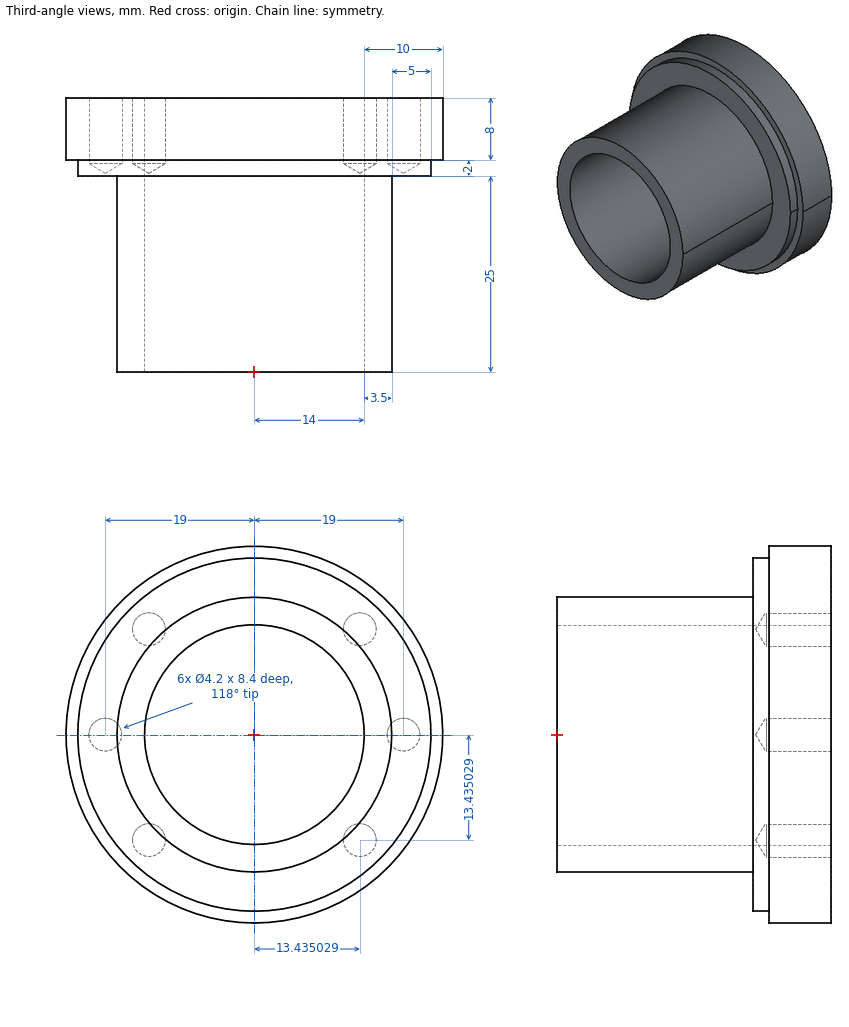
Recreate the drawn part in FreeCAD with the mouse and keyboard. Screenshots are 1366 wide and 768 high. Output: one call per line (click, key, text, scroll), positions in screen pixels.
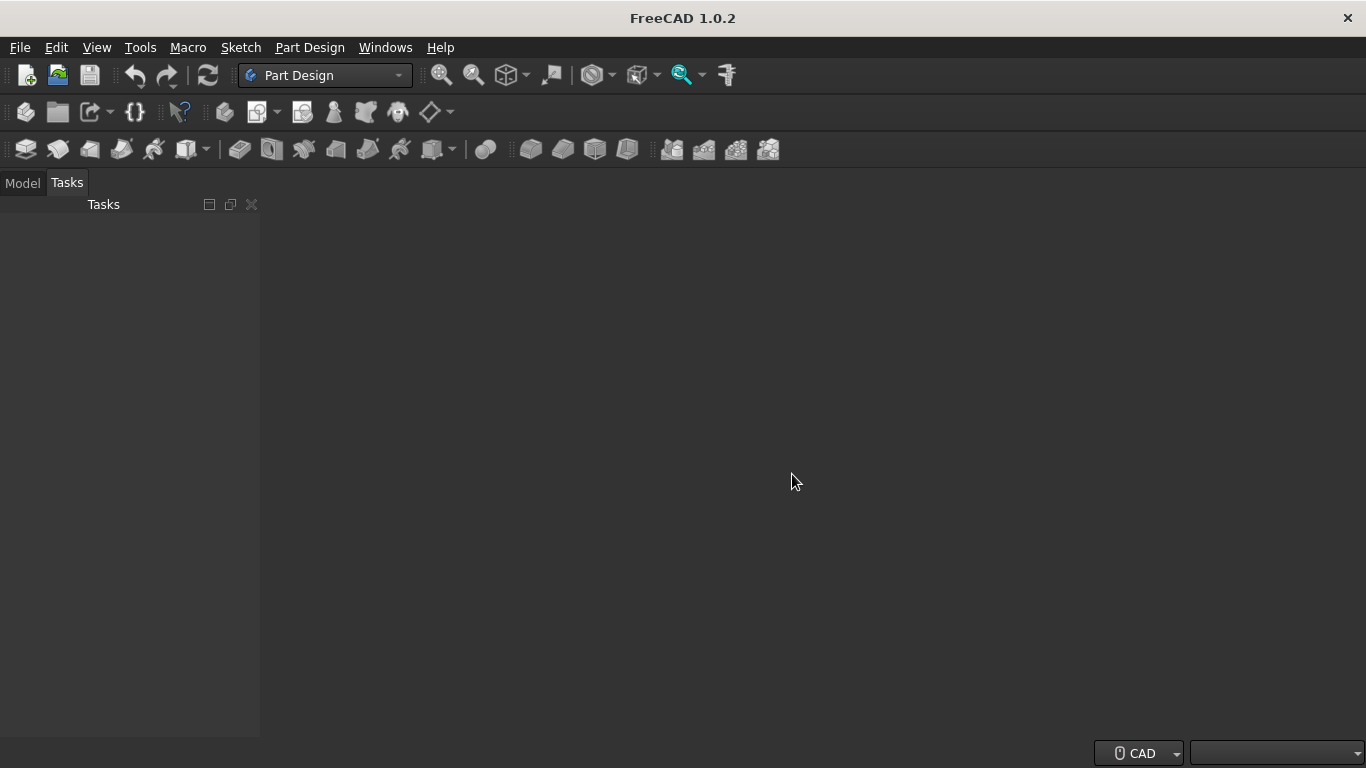
click(26, 76)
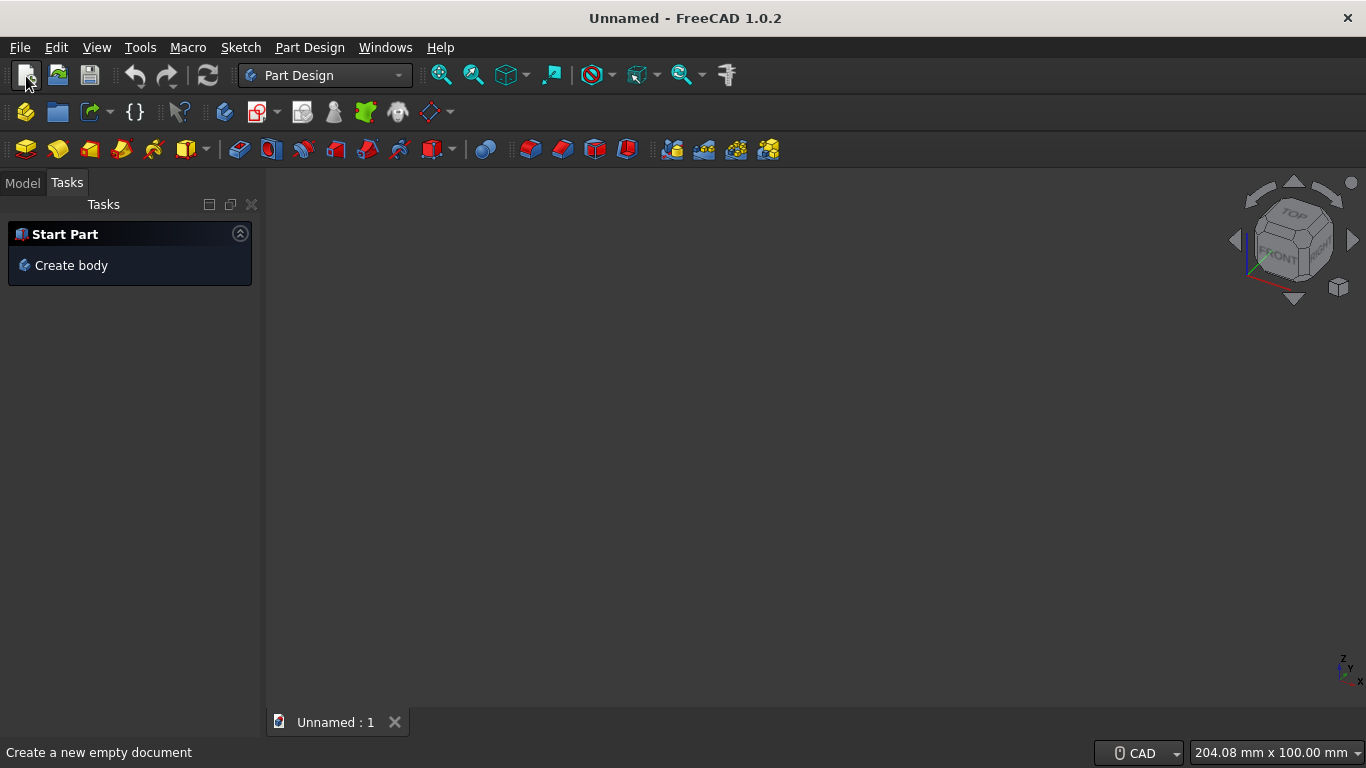
click(258, 112)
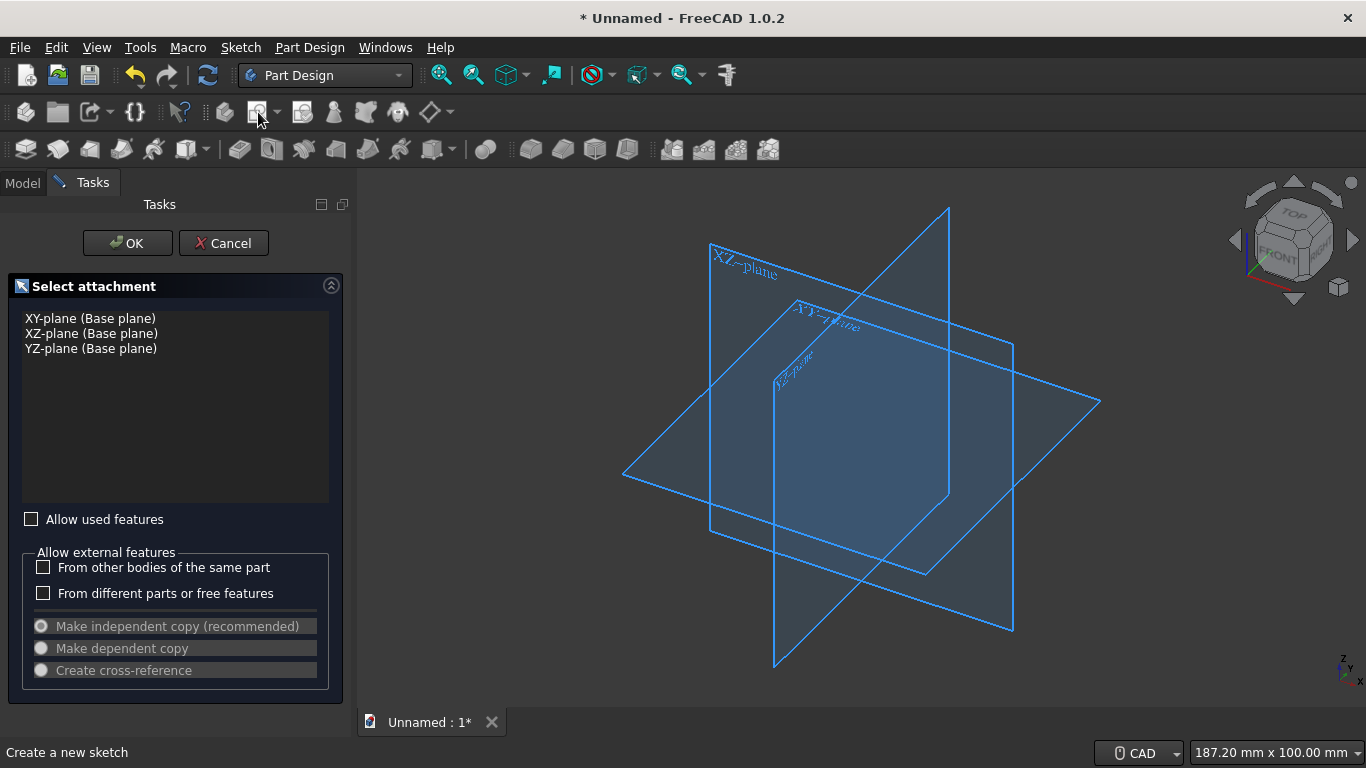
click(82, 318)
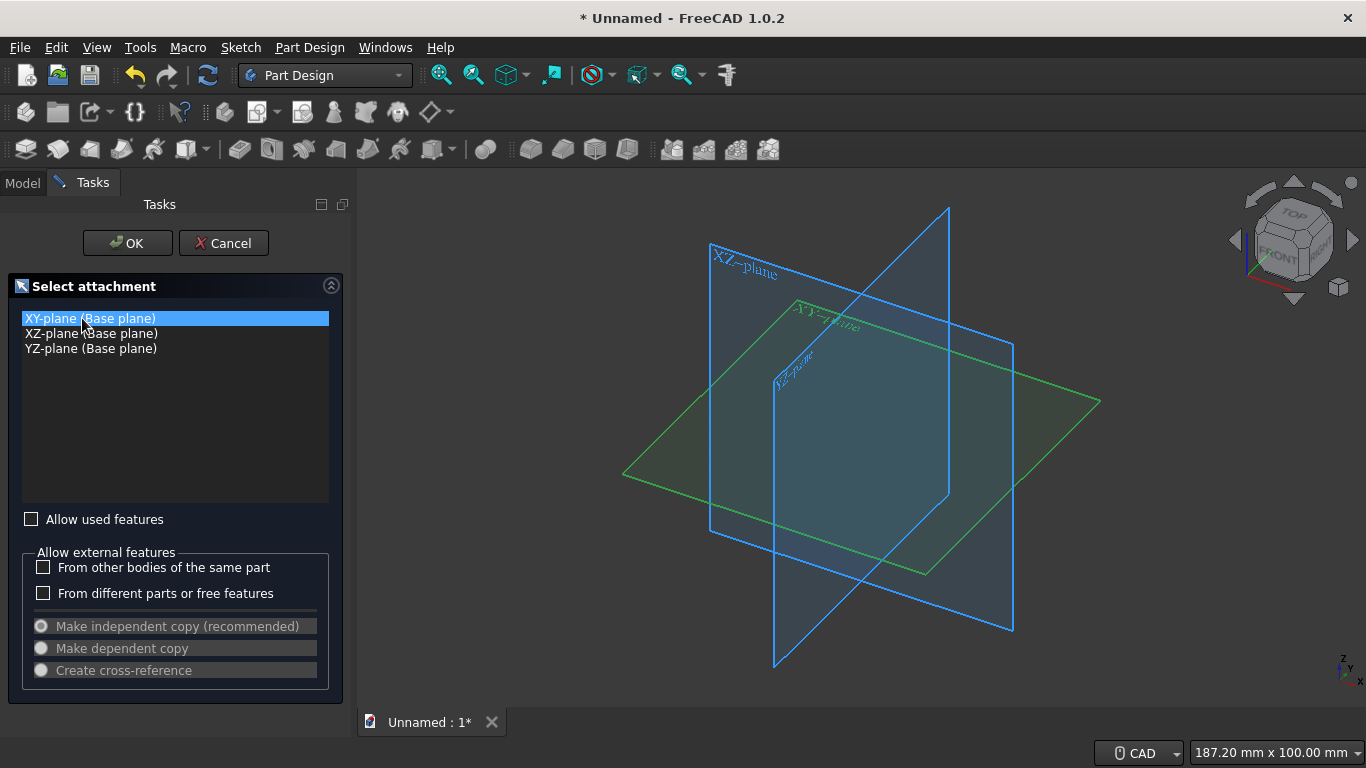
click(128, 243)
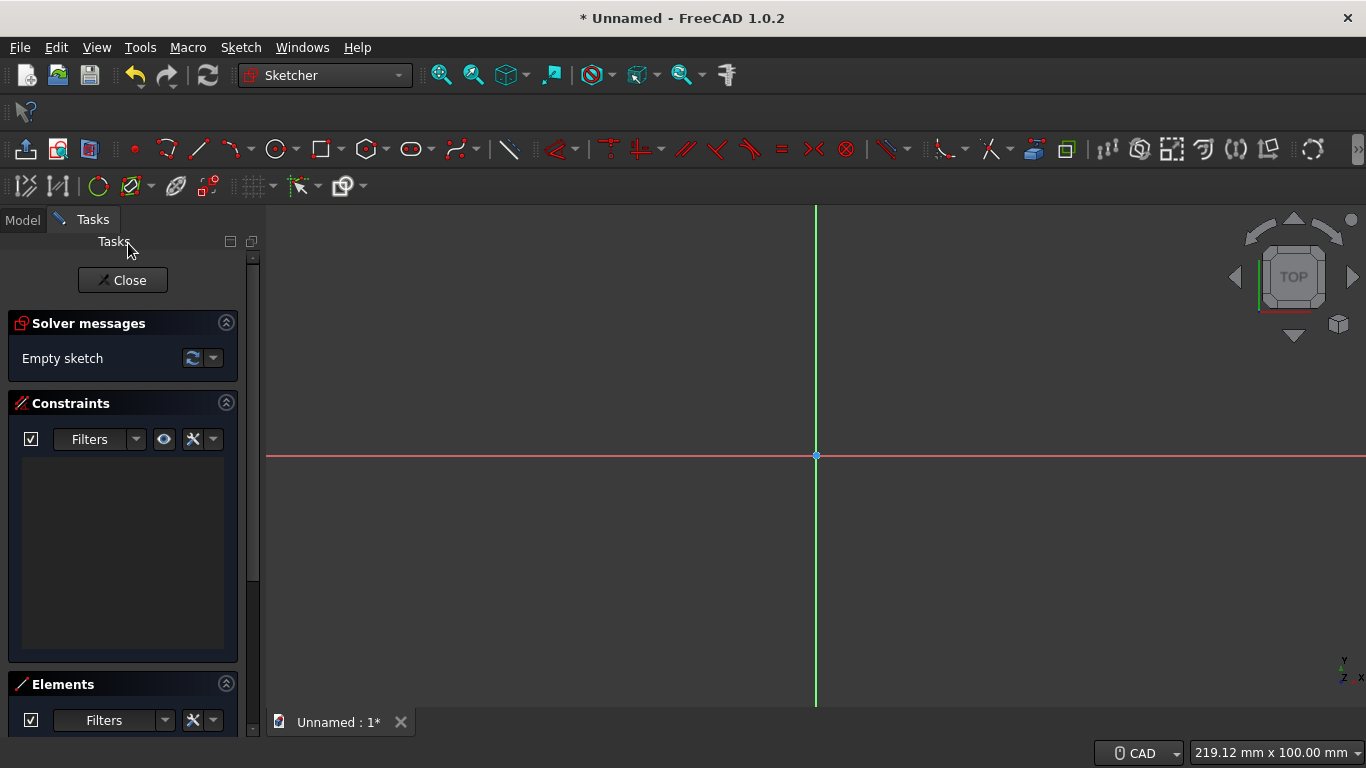
scroll(1033, 261, up, 3)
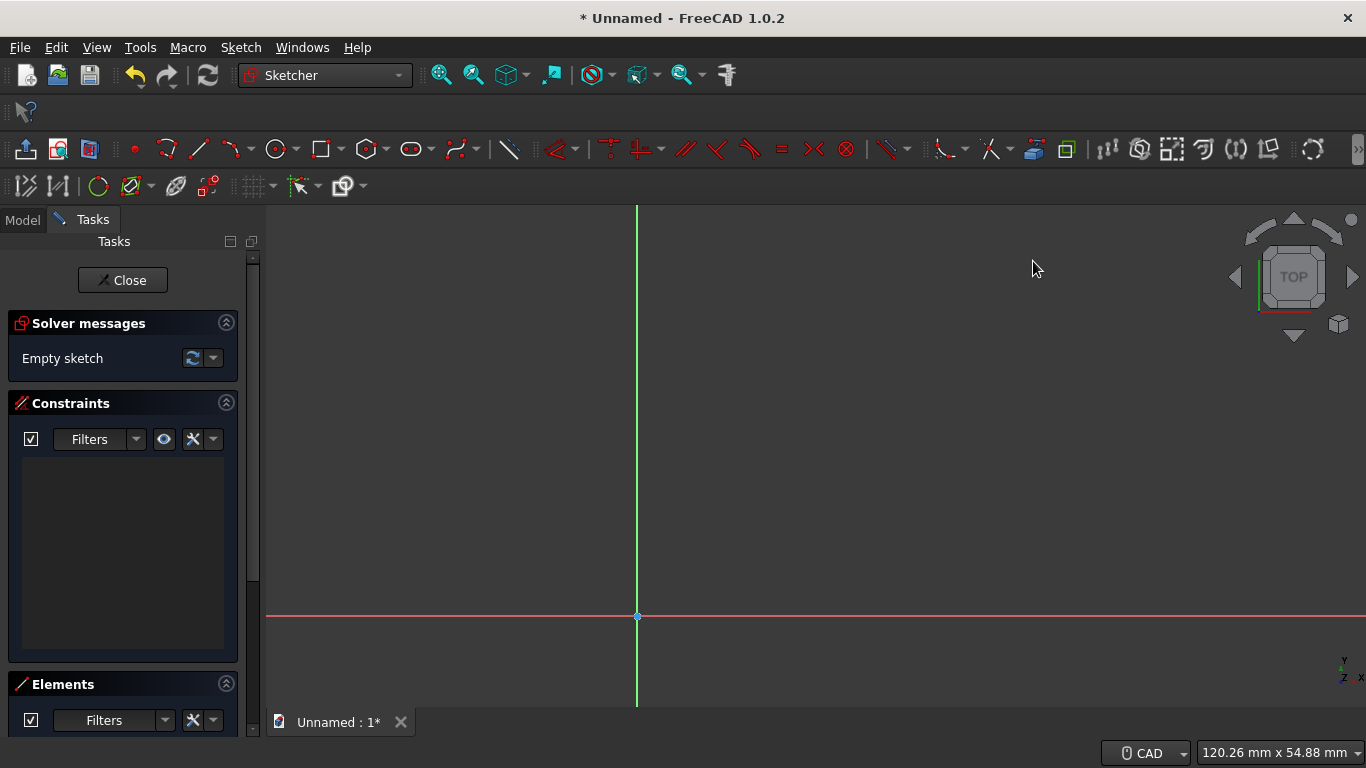
click(168, 150)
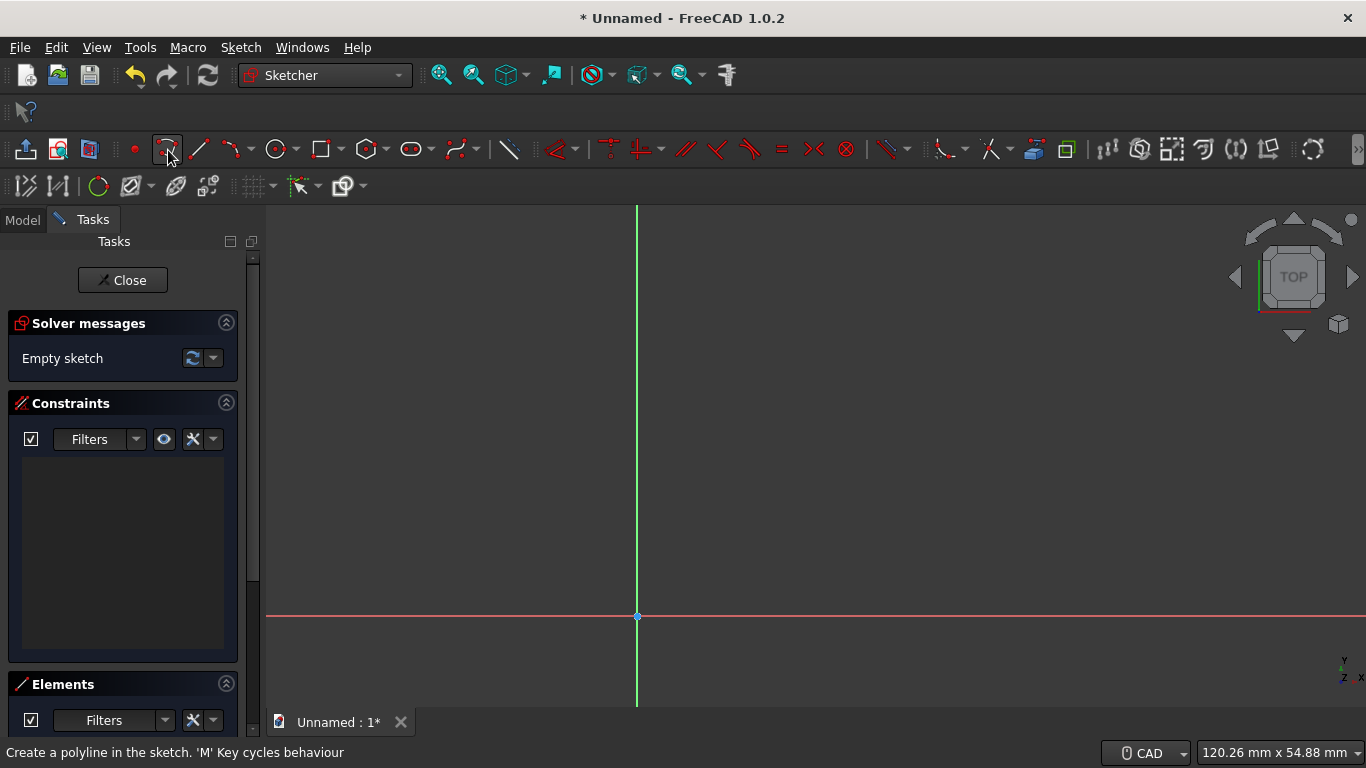
click(765, 616)
click(797, 607)
click(797, 388)
click(843, 388)
click(843, 369)
click(857, 369)
click(857, 296)
click(765, 296)
click(765, 616)
key(Escape)
key(Escape)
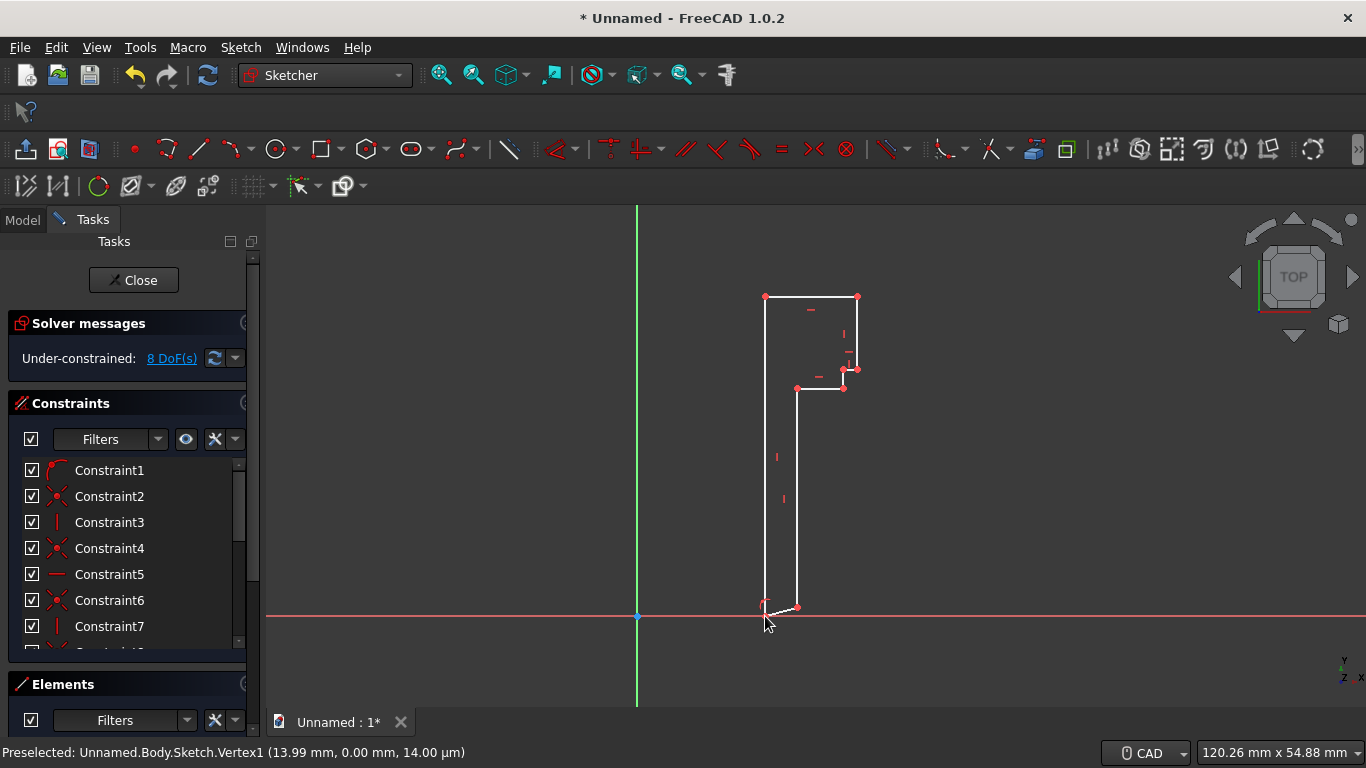
scroll(775, 614, up, 2)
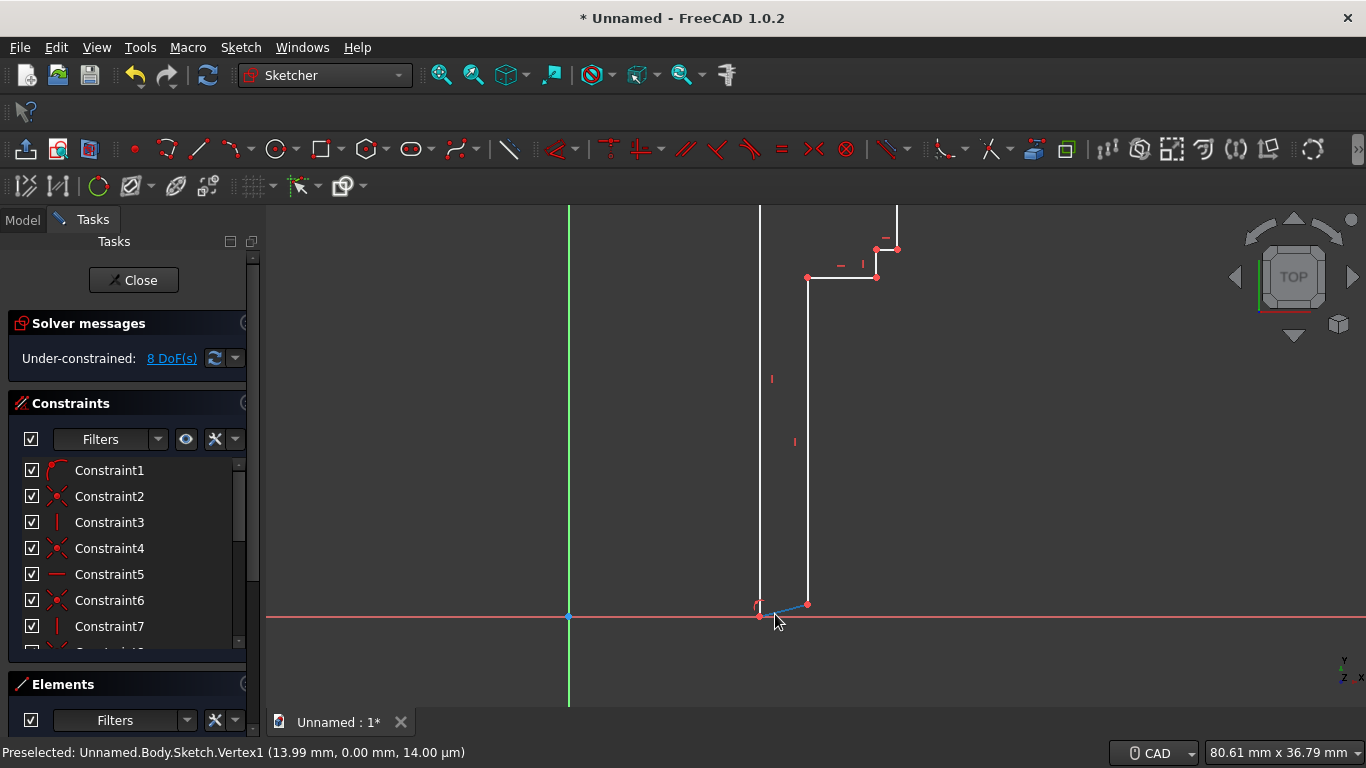
click(774, 613)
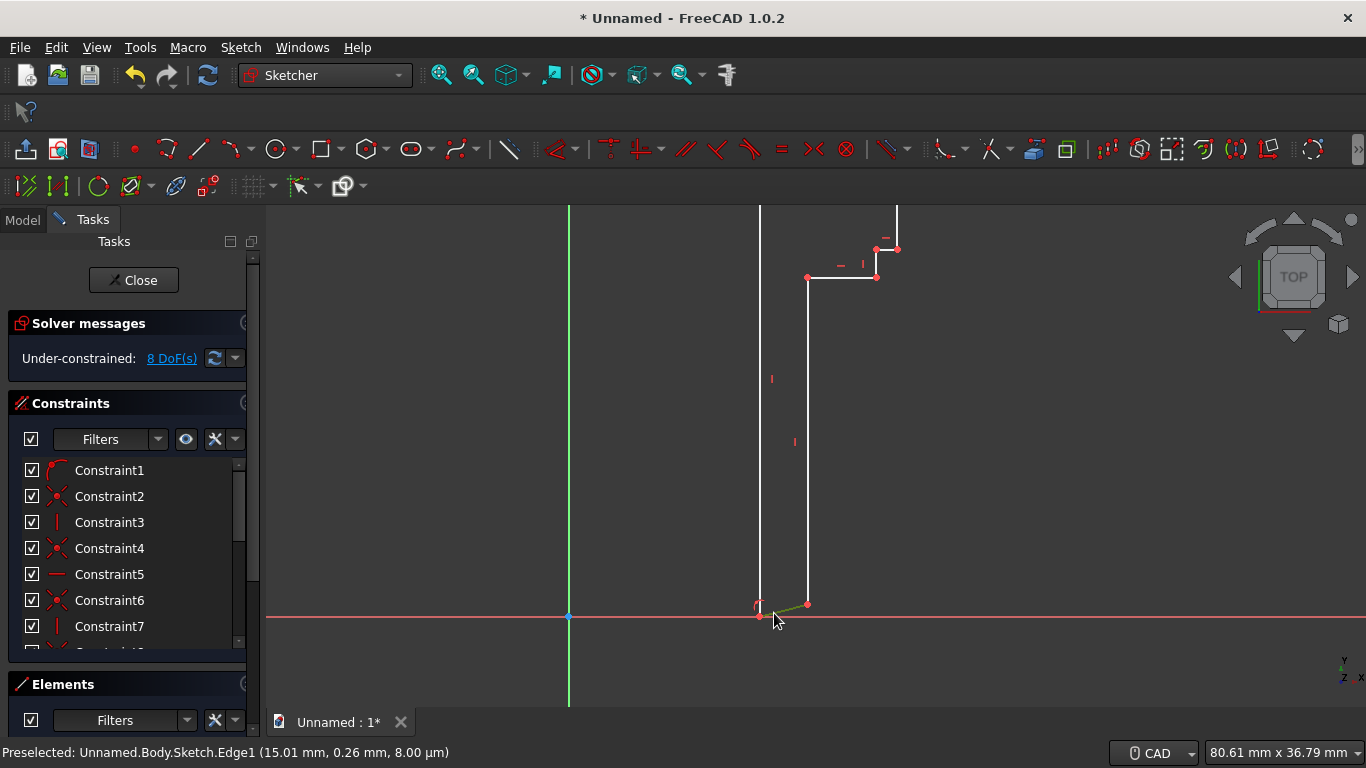
click(664, 150)